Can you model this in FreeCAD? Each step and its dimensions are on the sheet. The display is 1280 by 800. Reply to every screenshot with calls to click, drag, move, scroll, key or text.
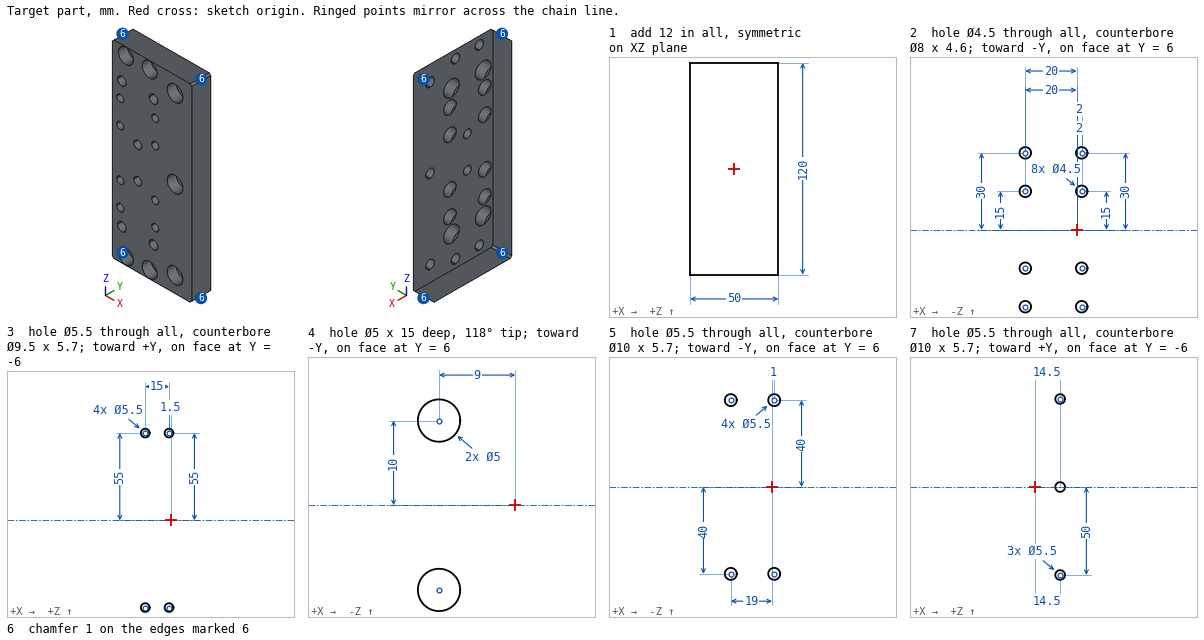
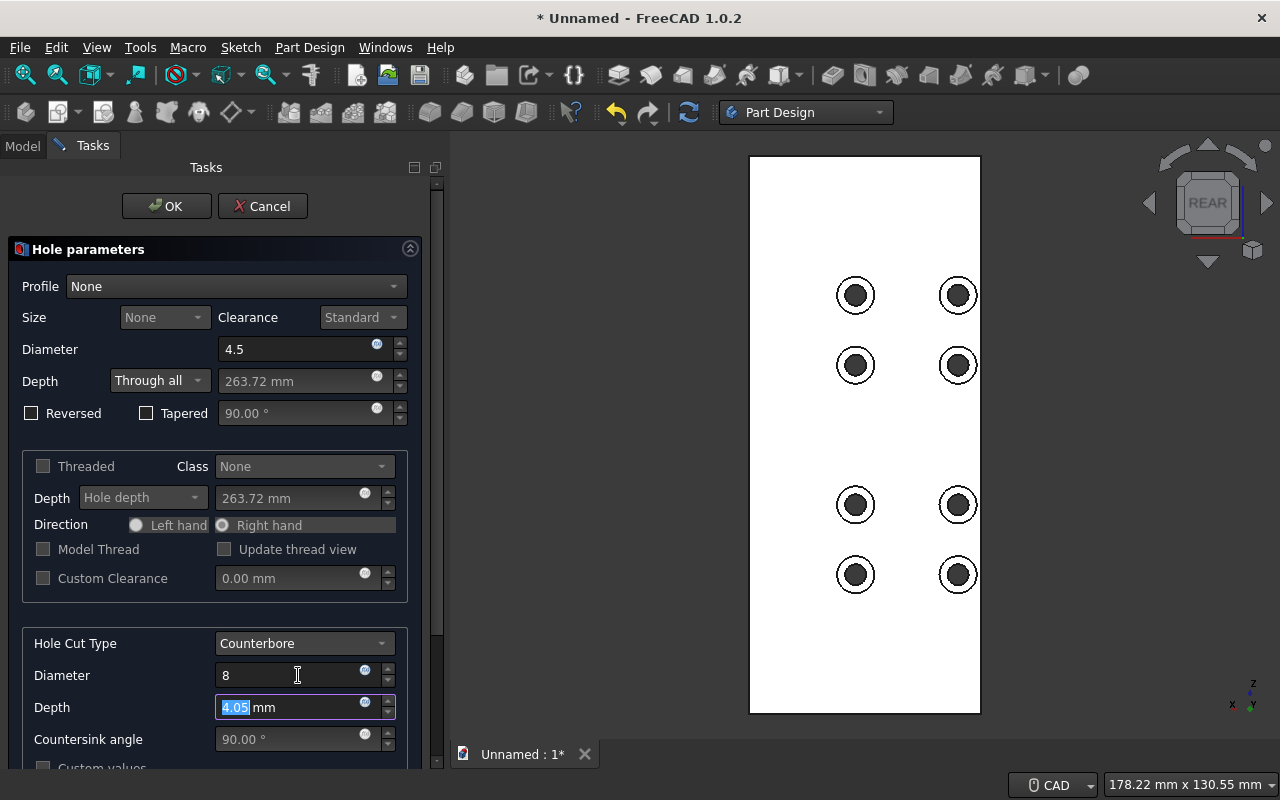
text(4.6)
key(Tab)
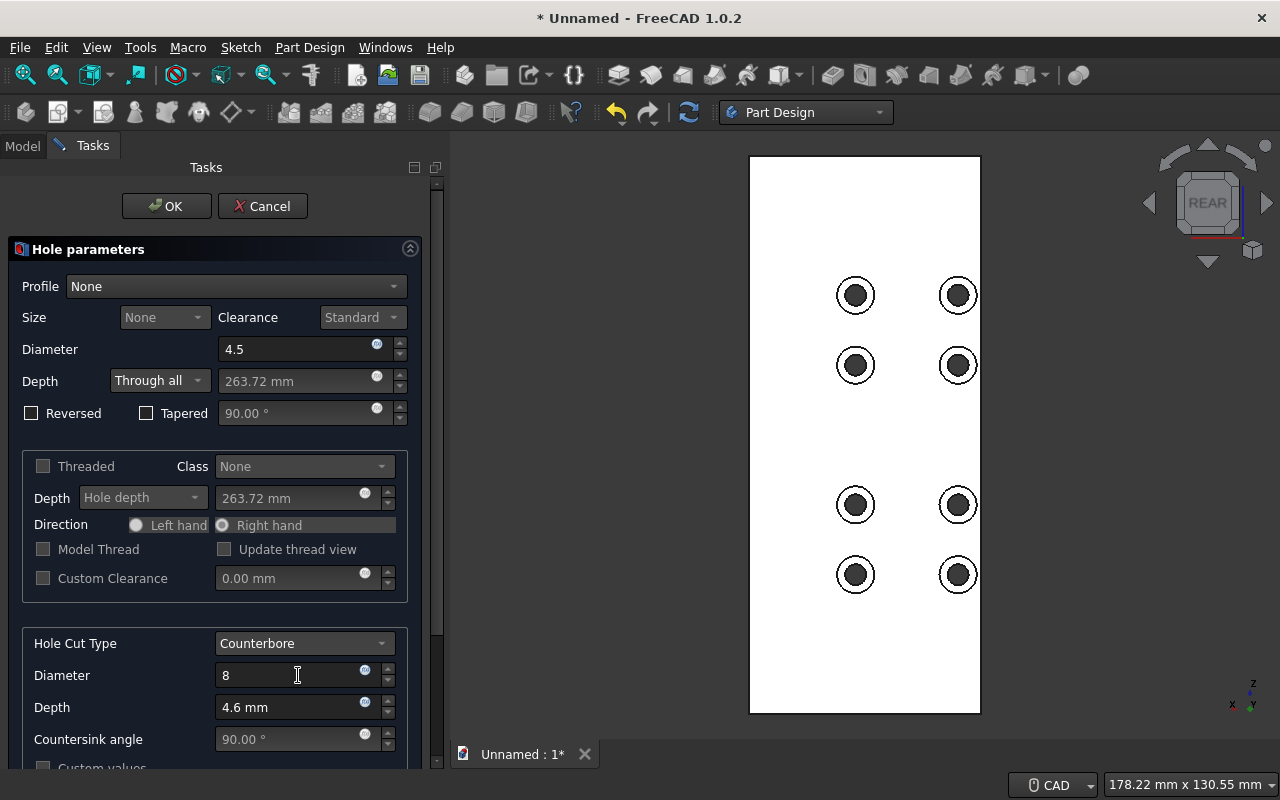
click(167, 206)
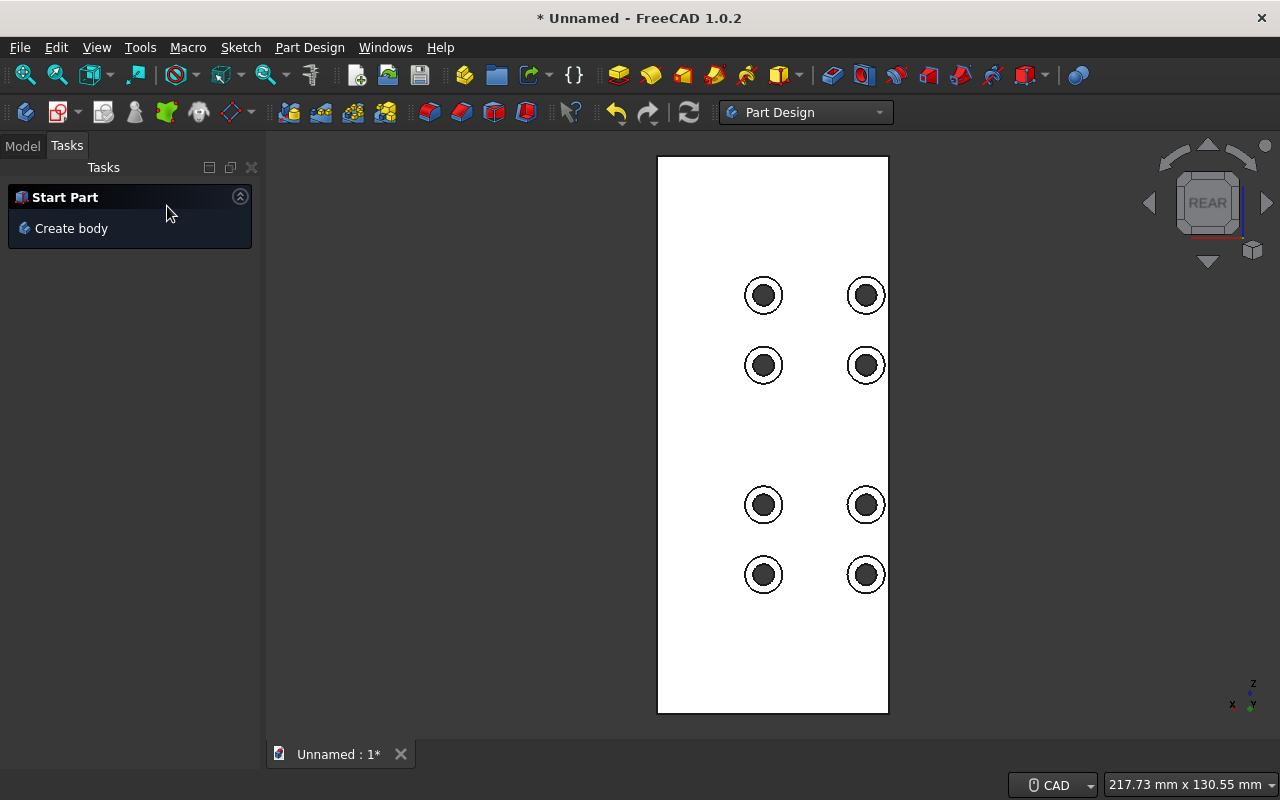
key(0)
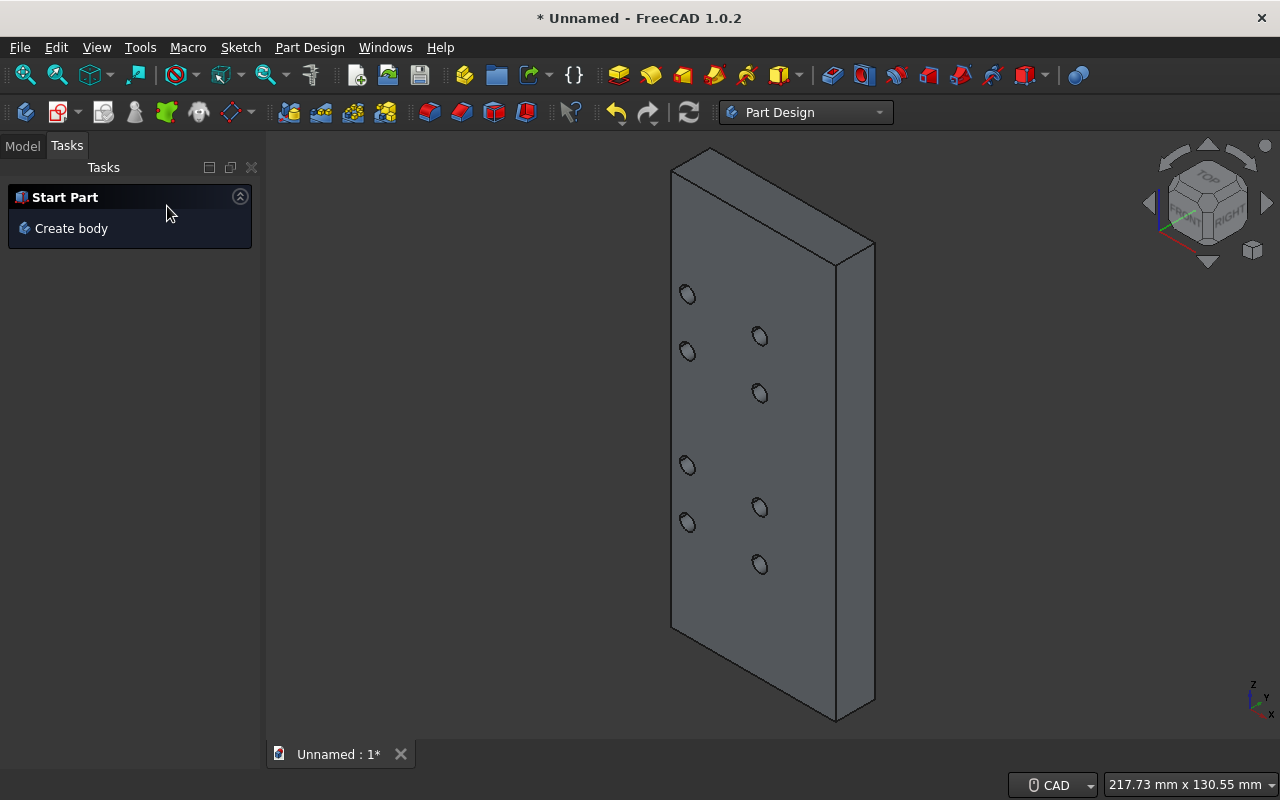
click(730, 432)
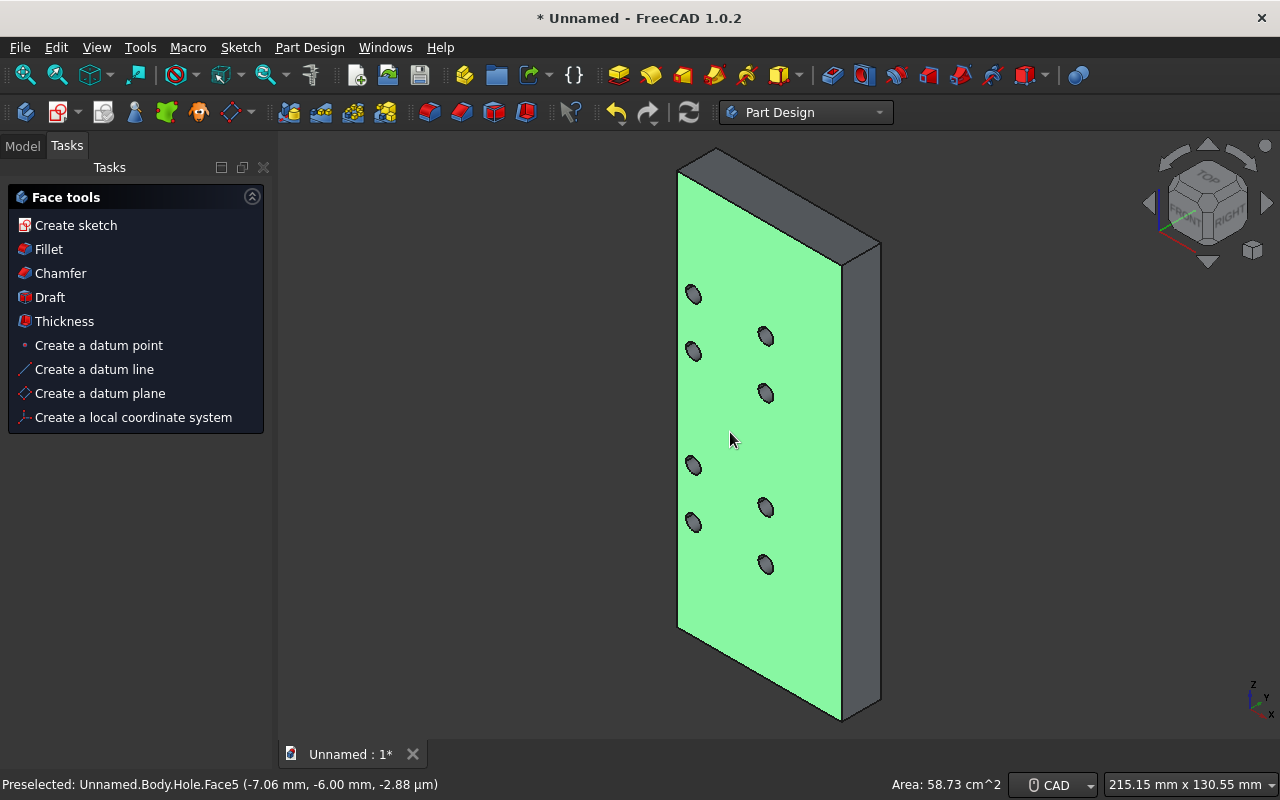
click(58, 112)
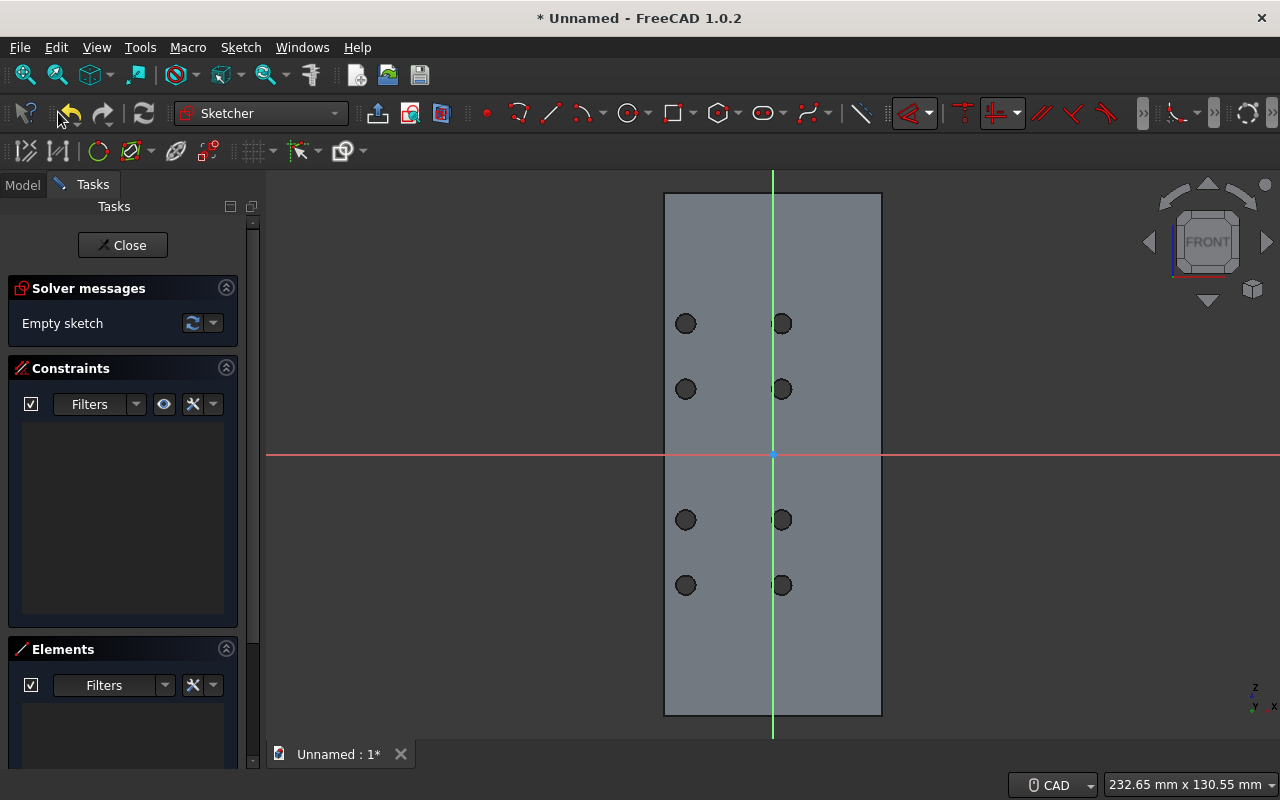
scroll(645, 454, down, 2)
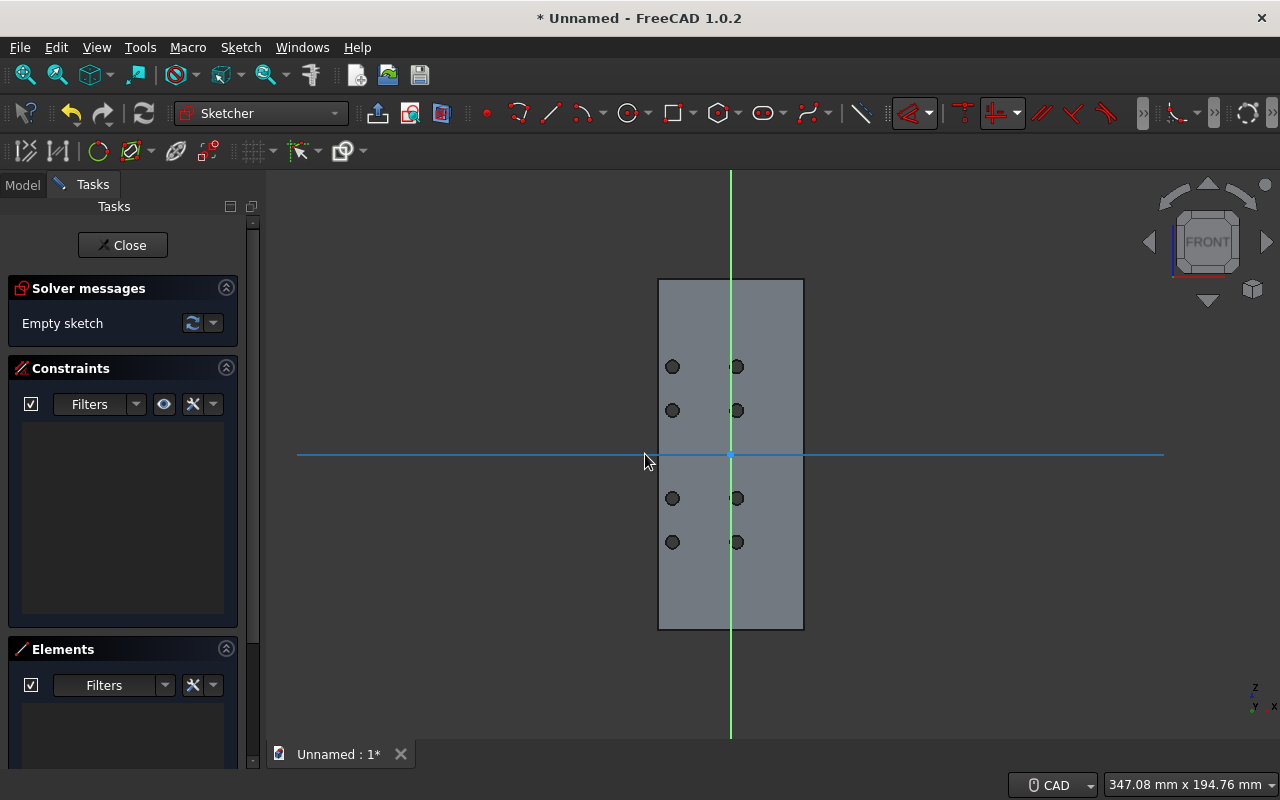
click(628, 114)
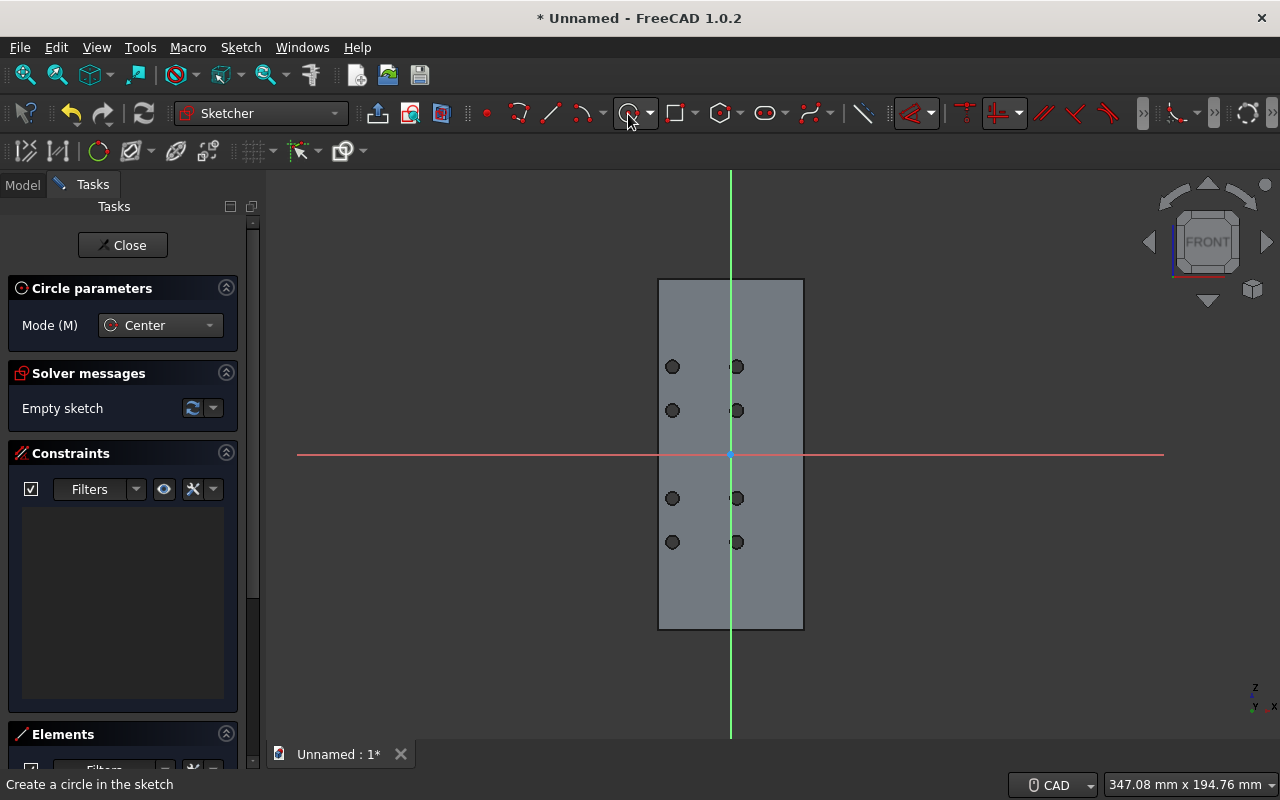
scroll(683, 294, up, 6)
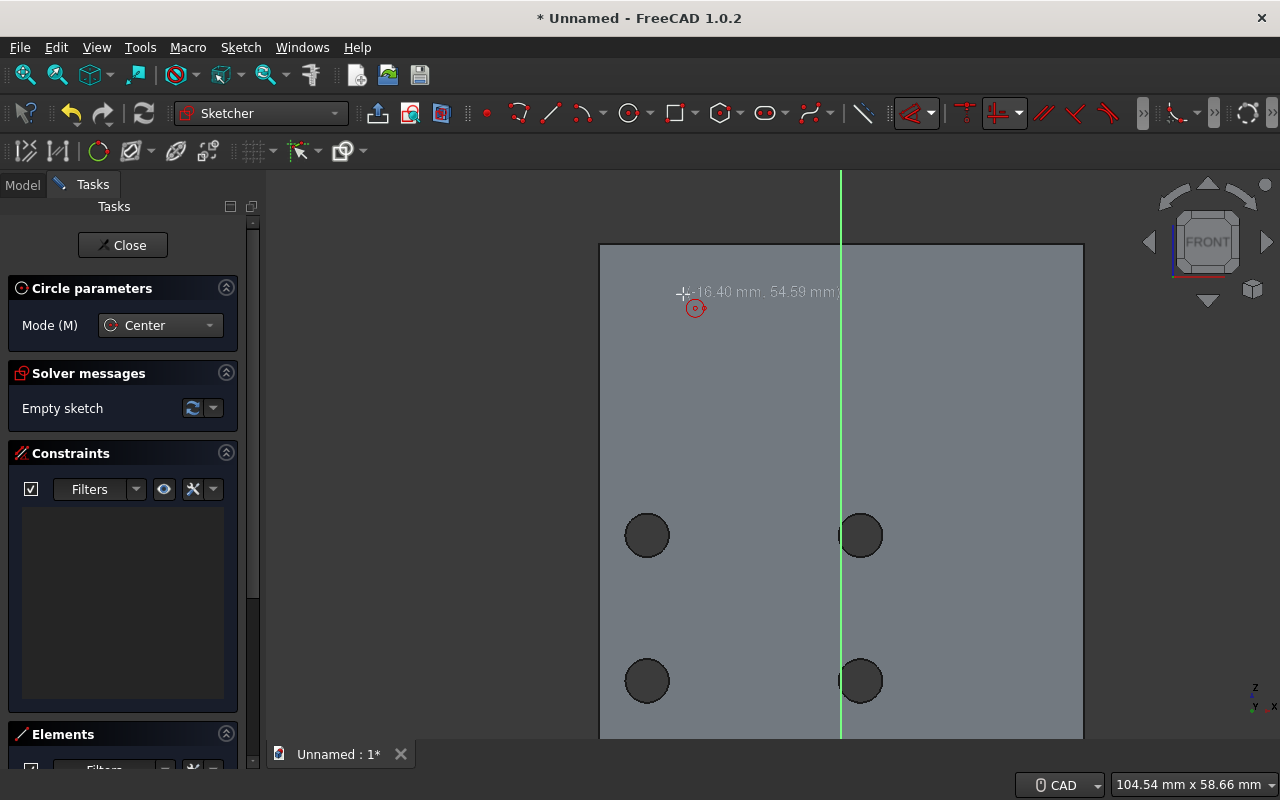
click(681, 293)
move(700, 274)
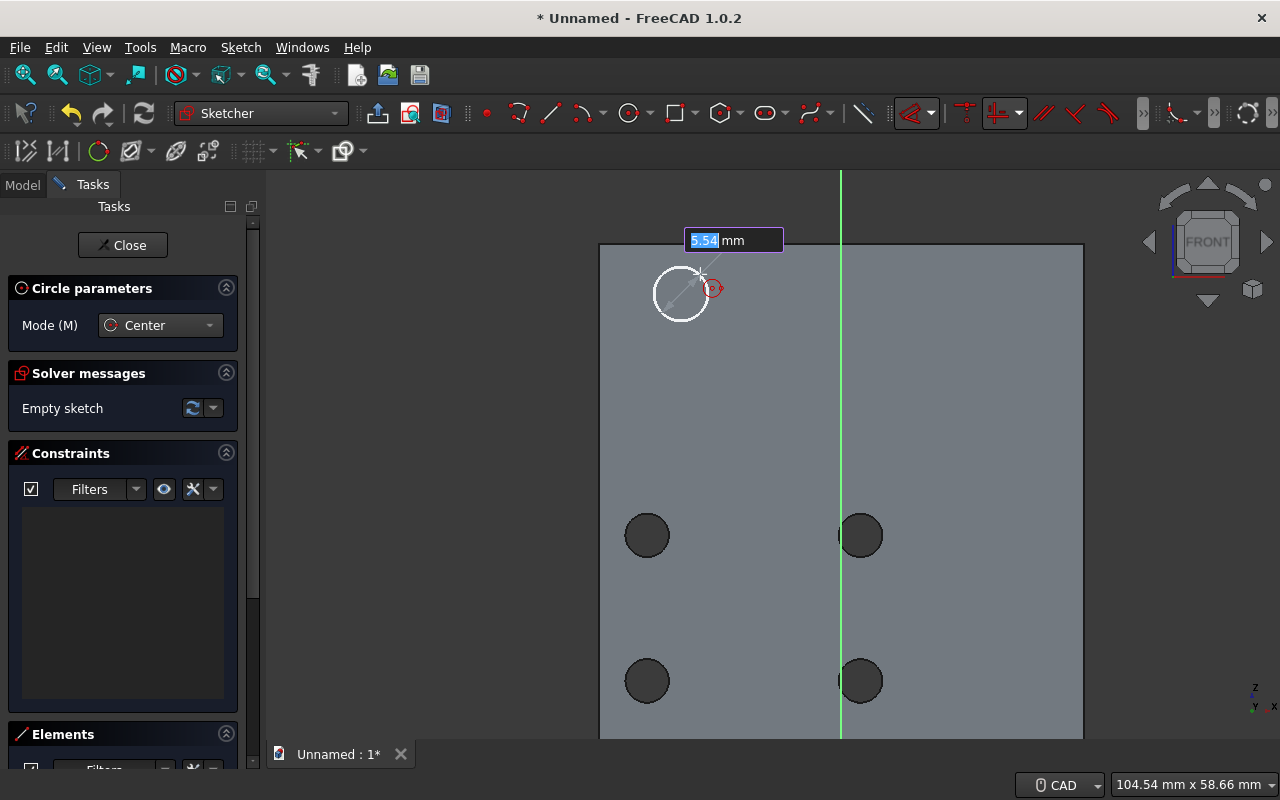
text(5.5)
key(Return)